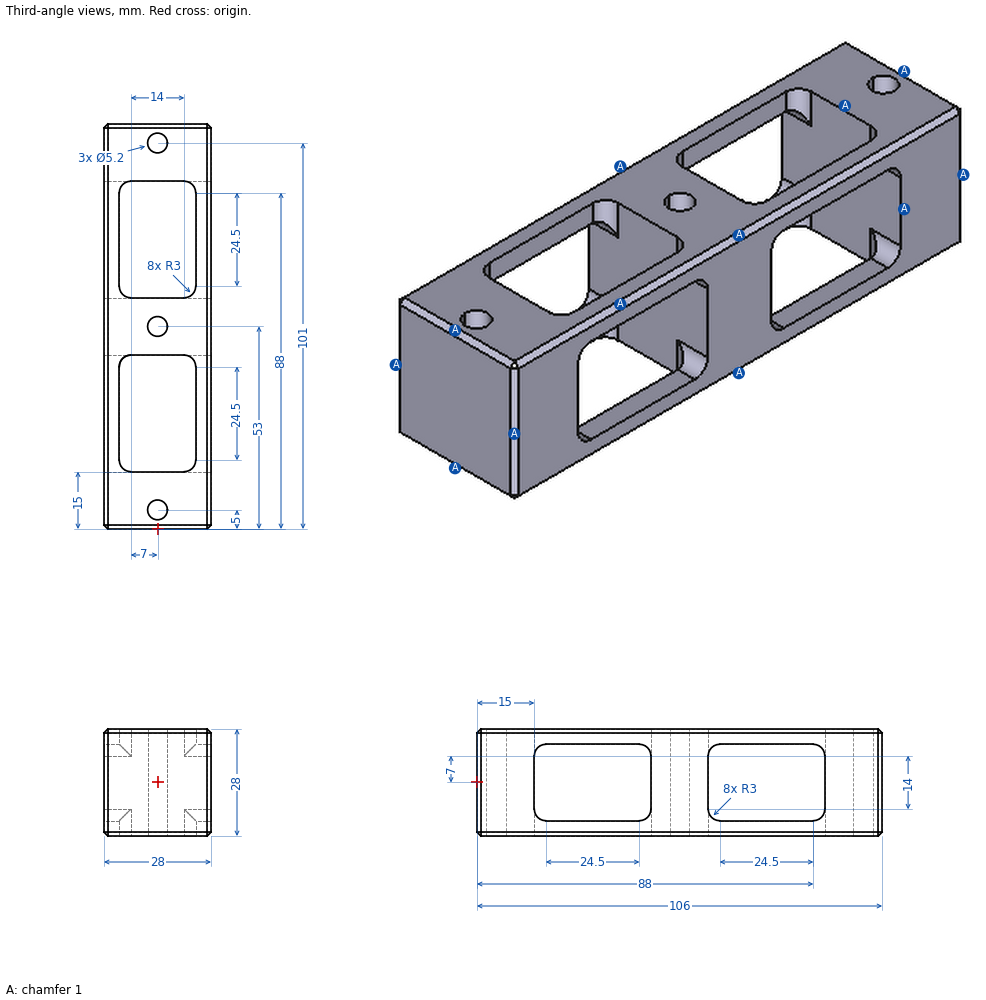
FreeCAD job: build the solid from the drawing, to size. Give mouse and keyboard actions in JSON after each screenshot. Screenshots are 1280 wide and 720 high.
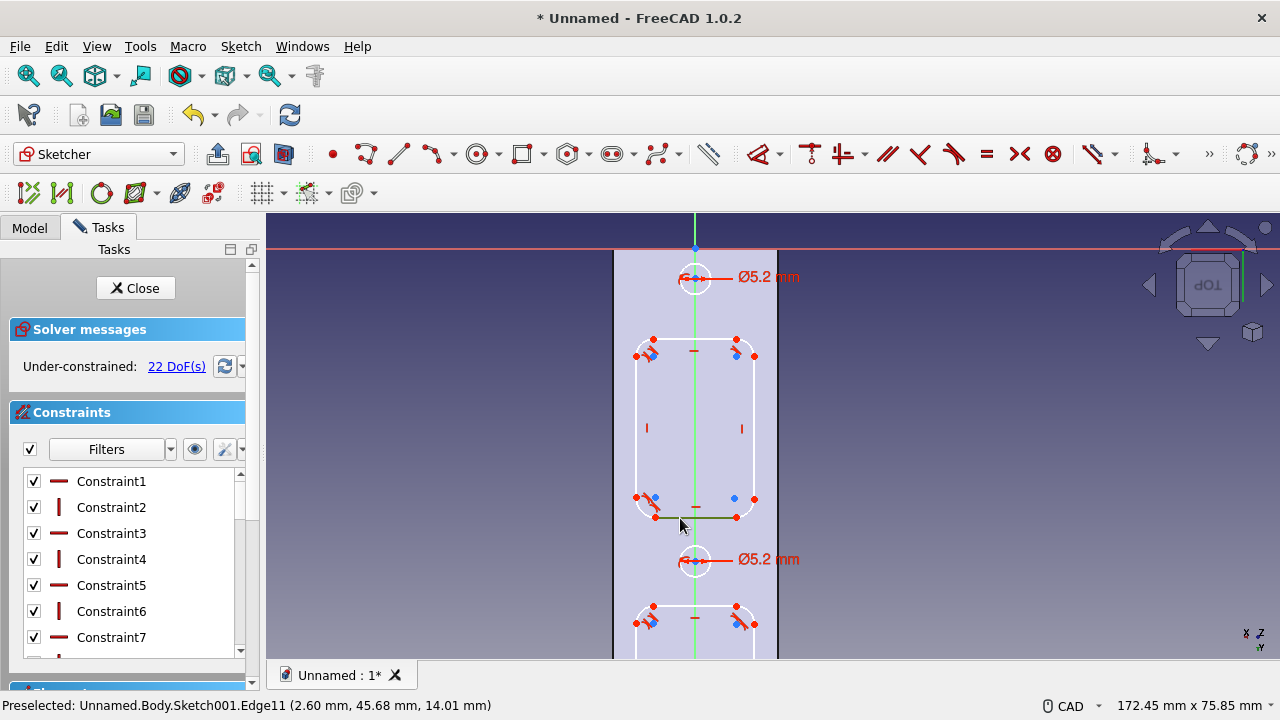
{"action": "left_click", "coordinate": [748, 512]}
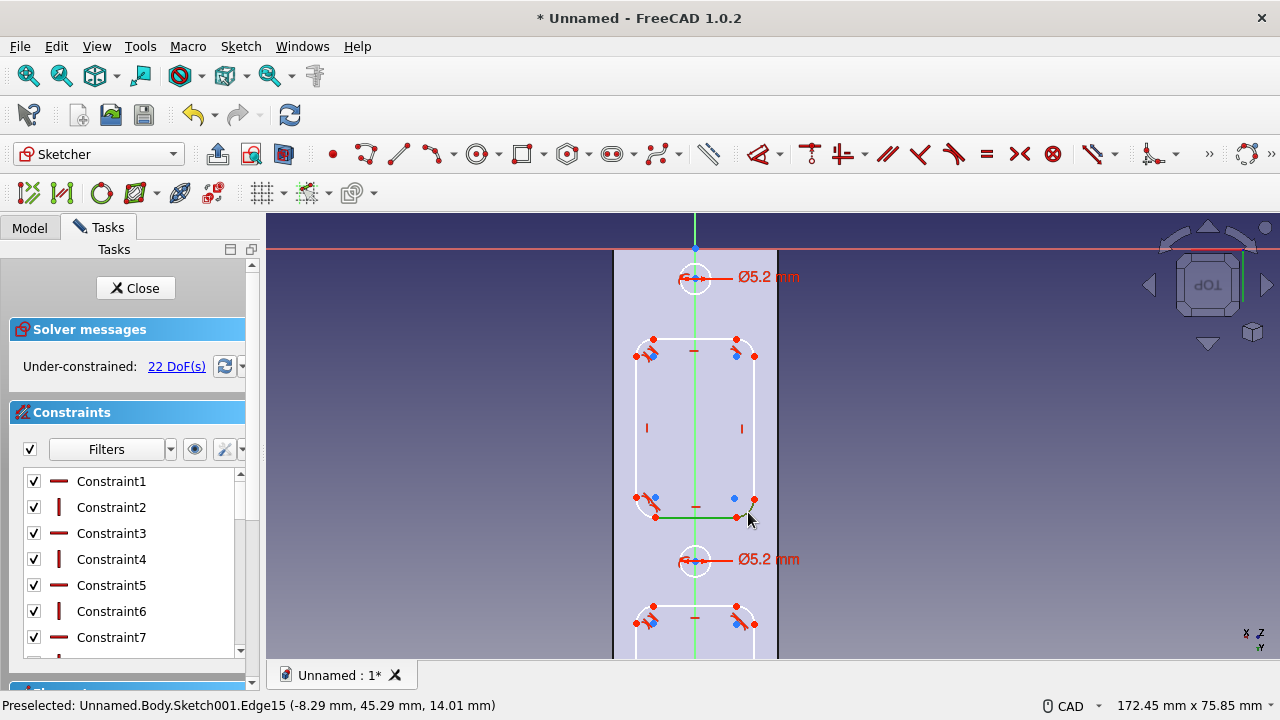
{"action": "left_click", "coordinate": [954, 154]}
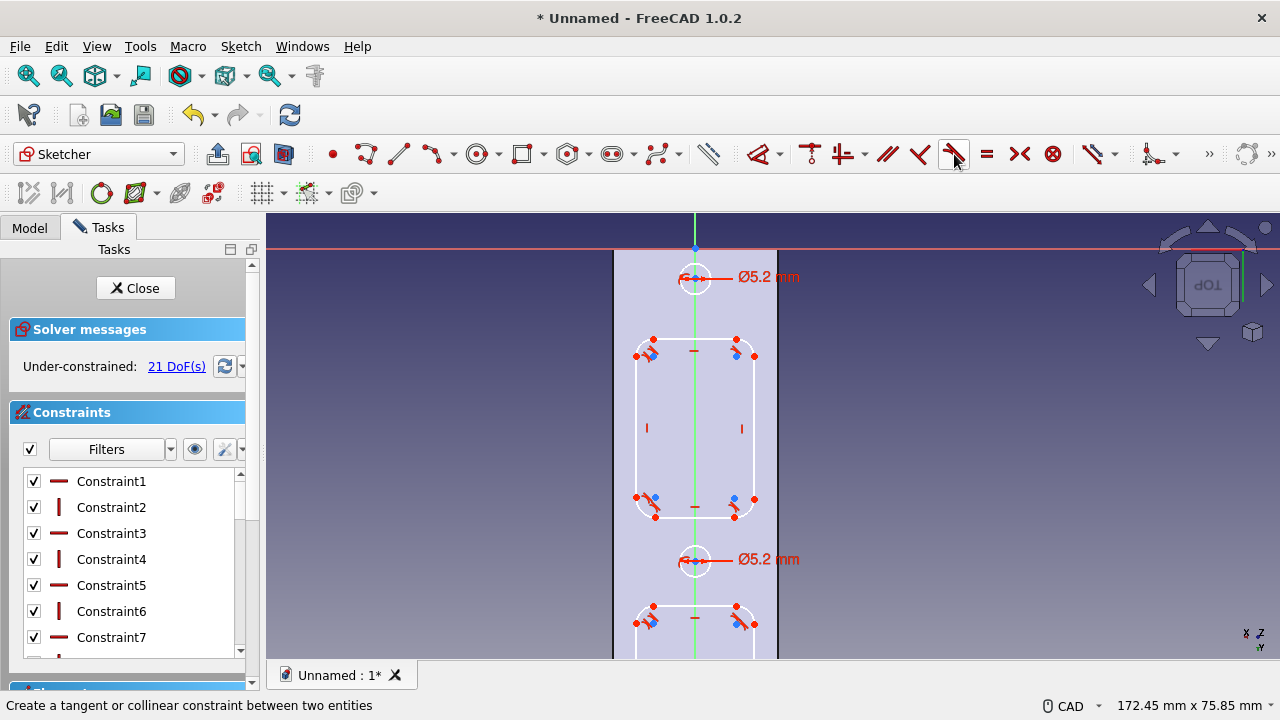
{"action": "left_click", "coordinate": [754, 457]}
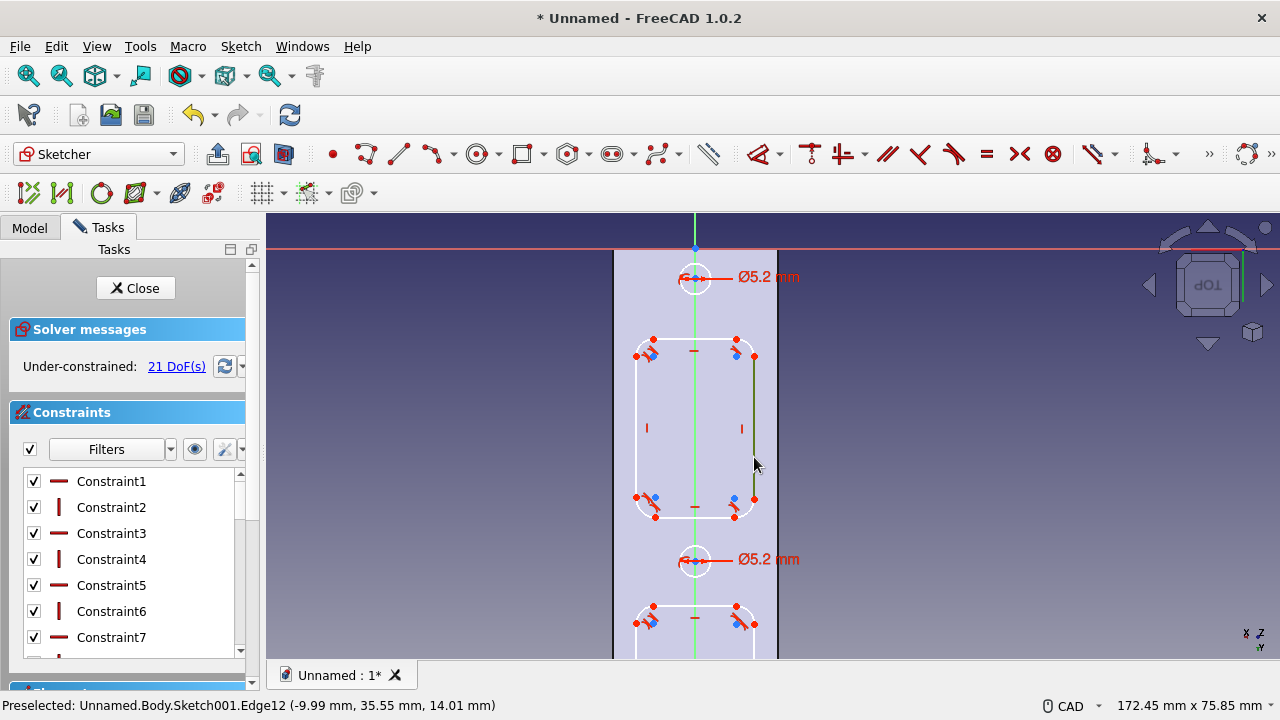
{"action": "left_click", "coordinate": [748, 512]}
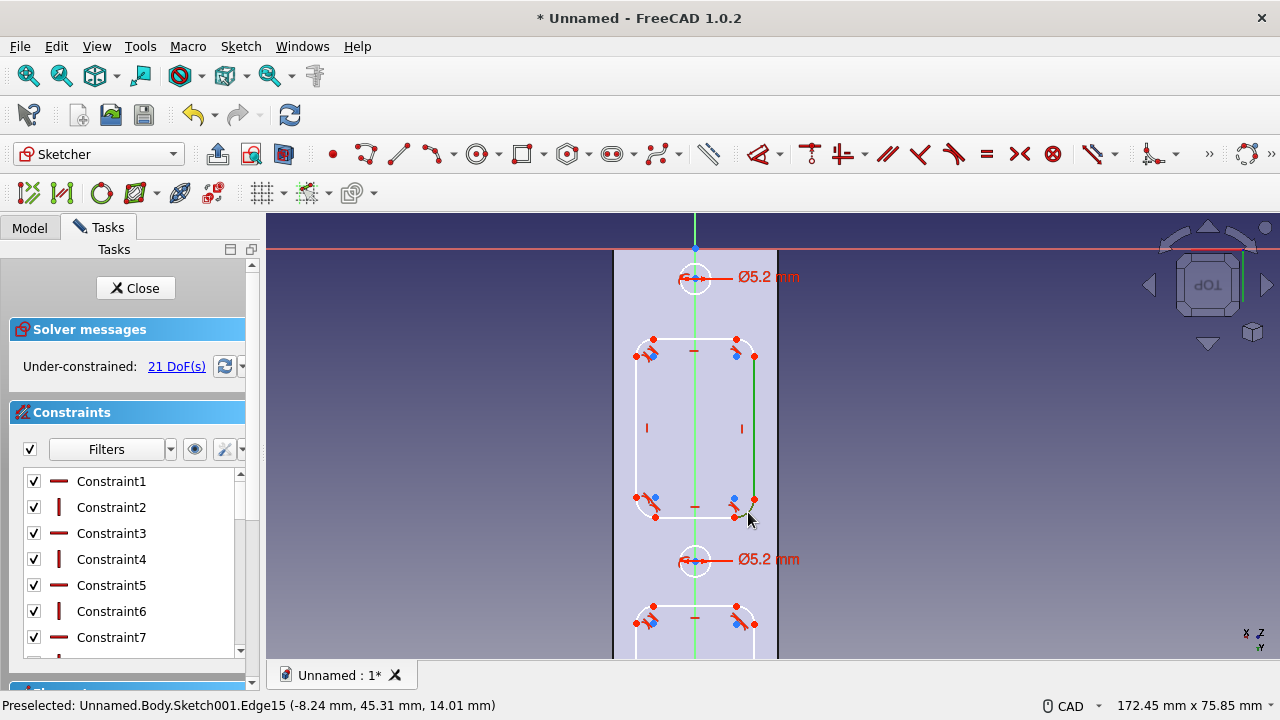
{"action": "left_click", "coordinate": [954, 154]}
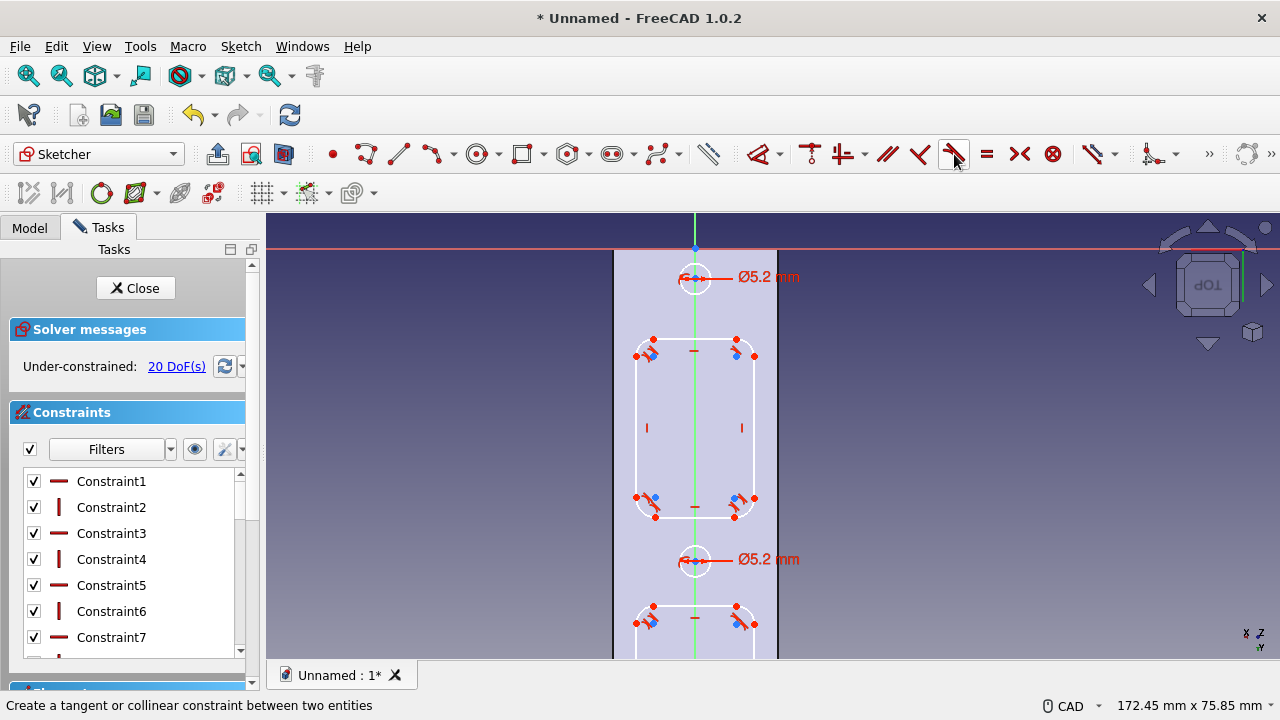
{"action": "left_click", "coordinate": [754, 456]}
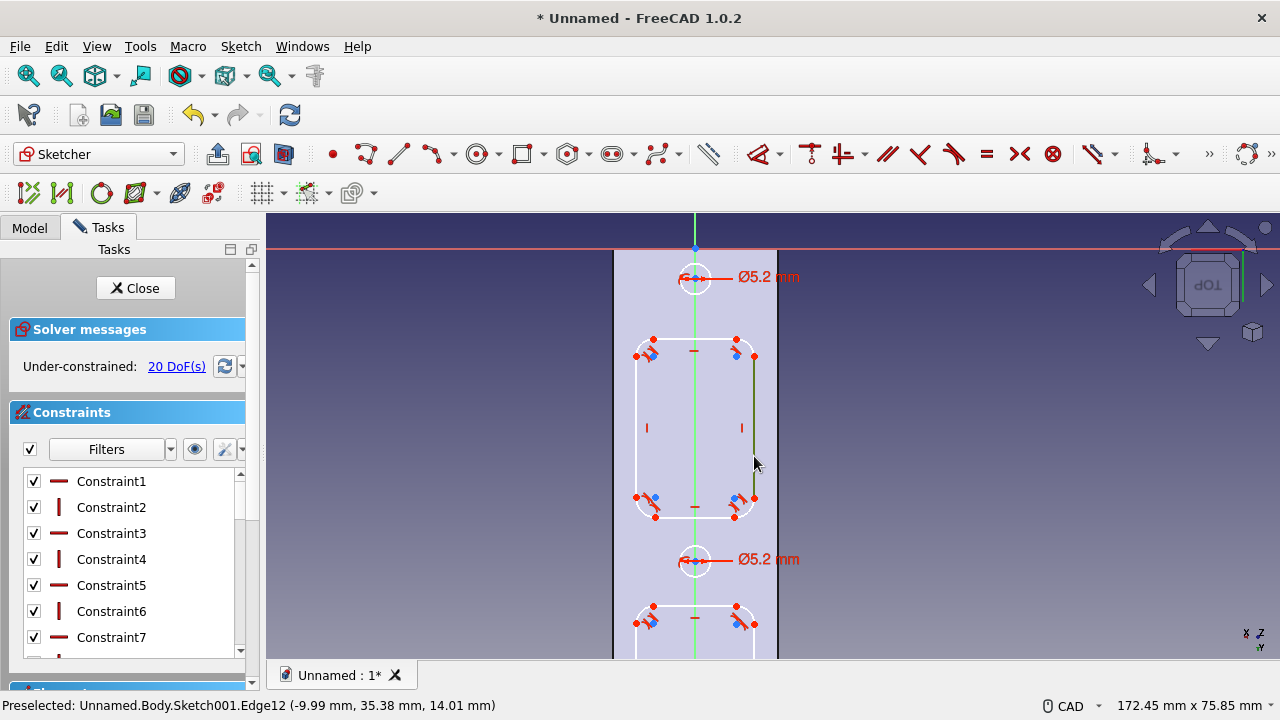
{"action": "left_click", "coordinate": [749, 344]}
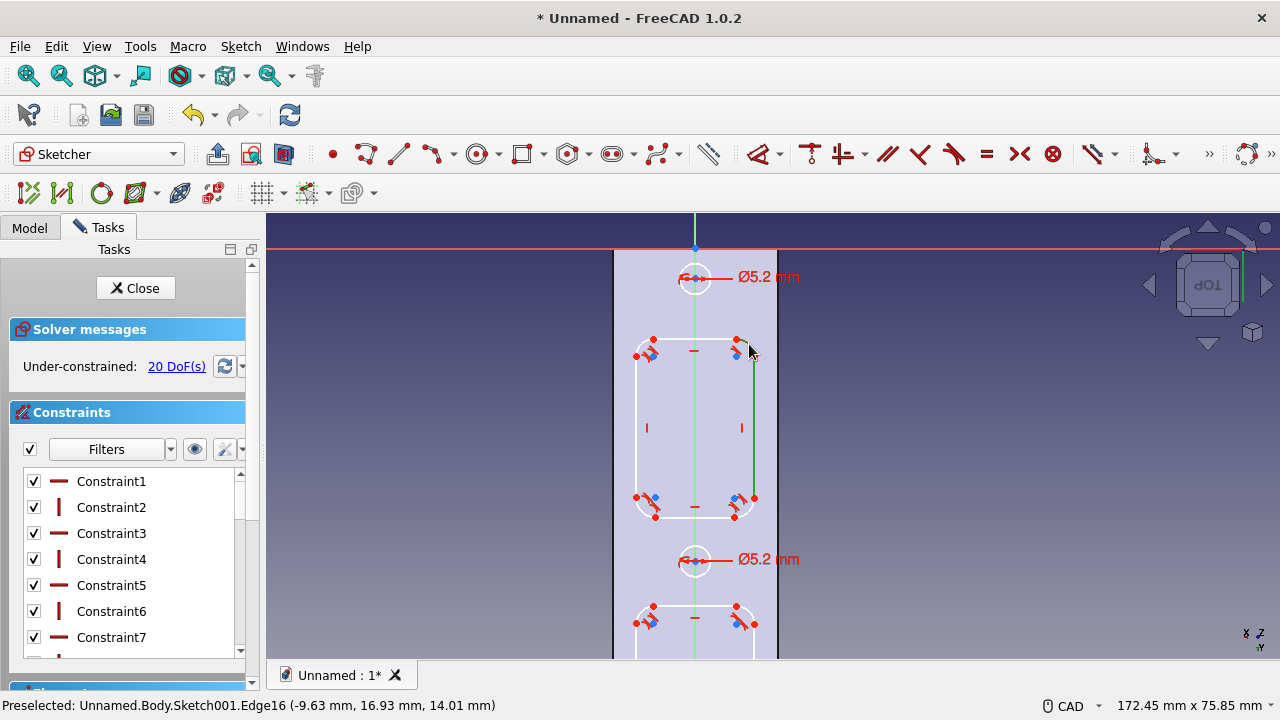
{"action": "left_click", "coordinate": [954, 154]}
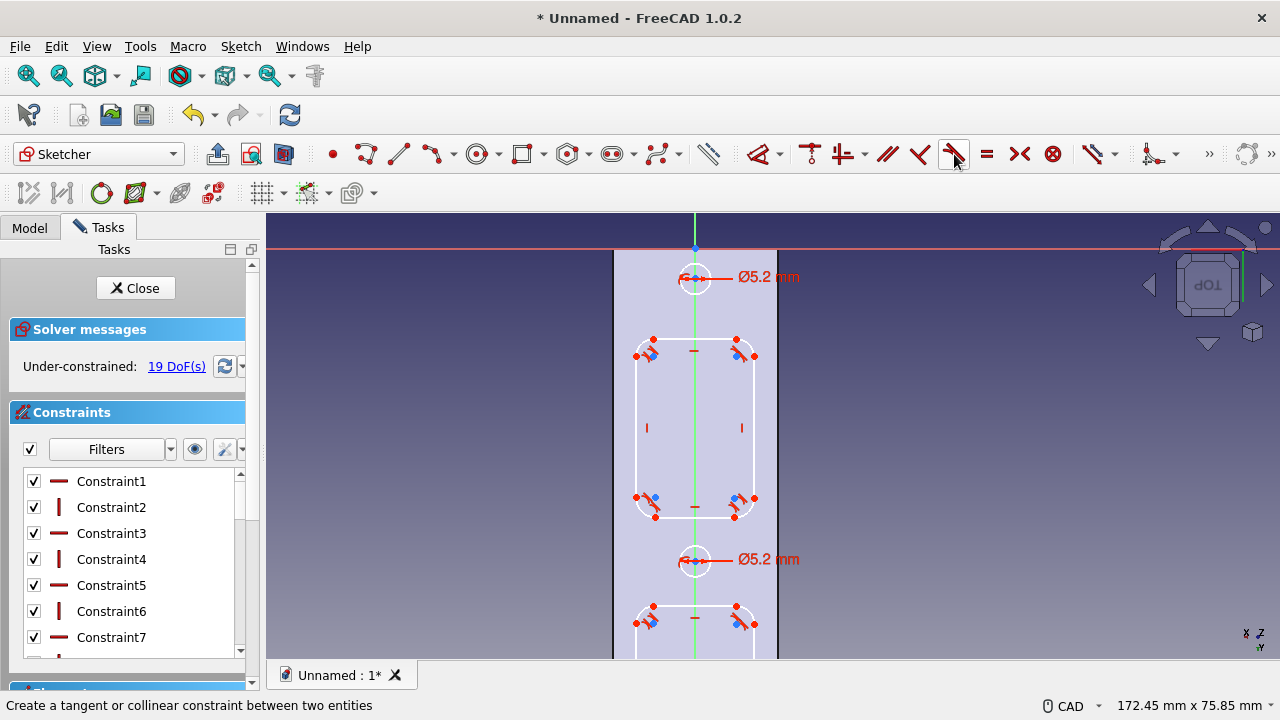
{"action": "left_click", "coordinate": [642, 611]}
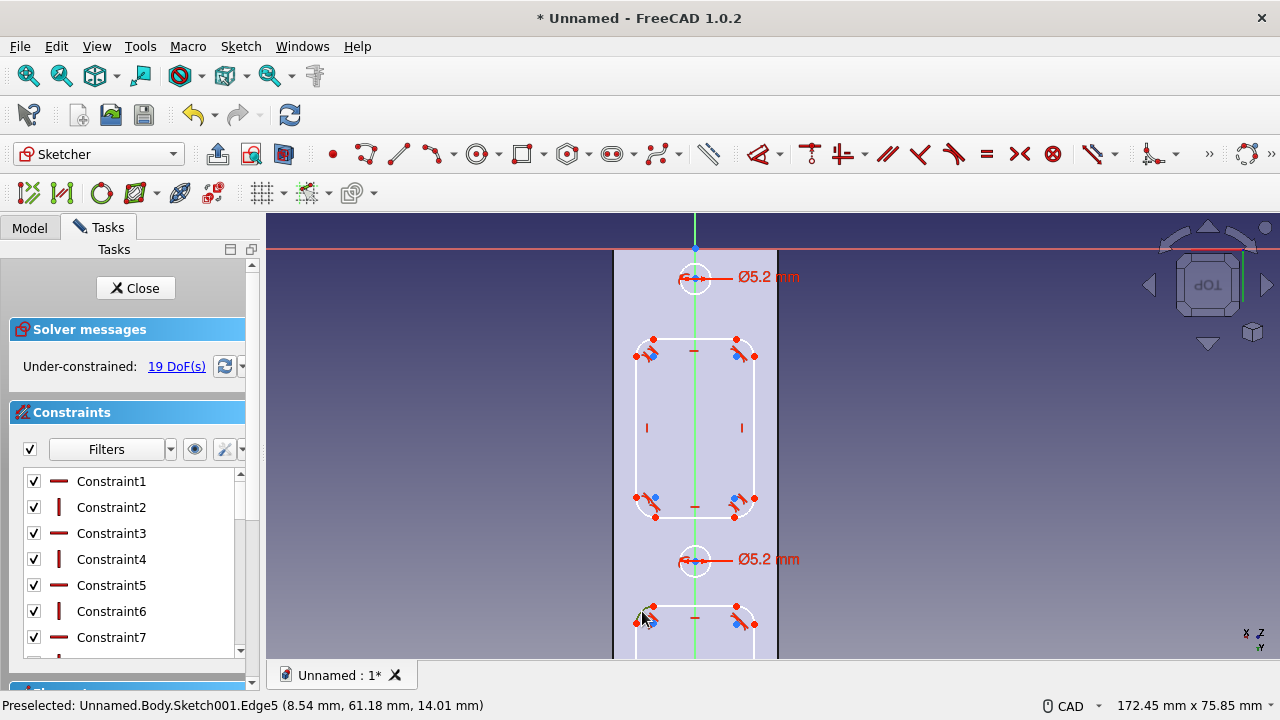
{"action": "scroll", "coordinate": [712, 340], "scroll_direction": "down", "scroll_amount": 4}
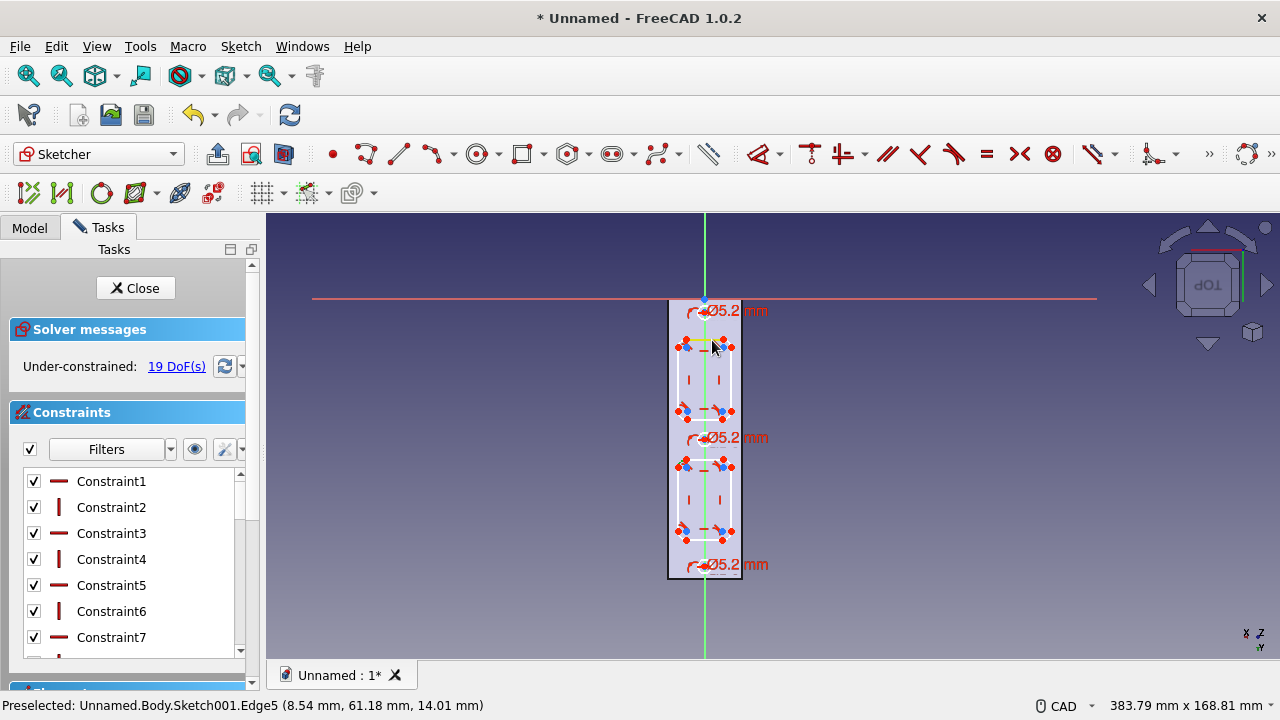
{"action": "scroll", "coordinate": [681, 538], "scroll_direction": "up", "scroll_amount": 4}